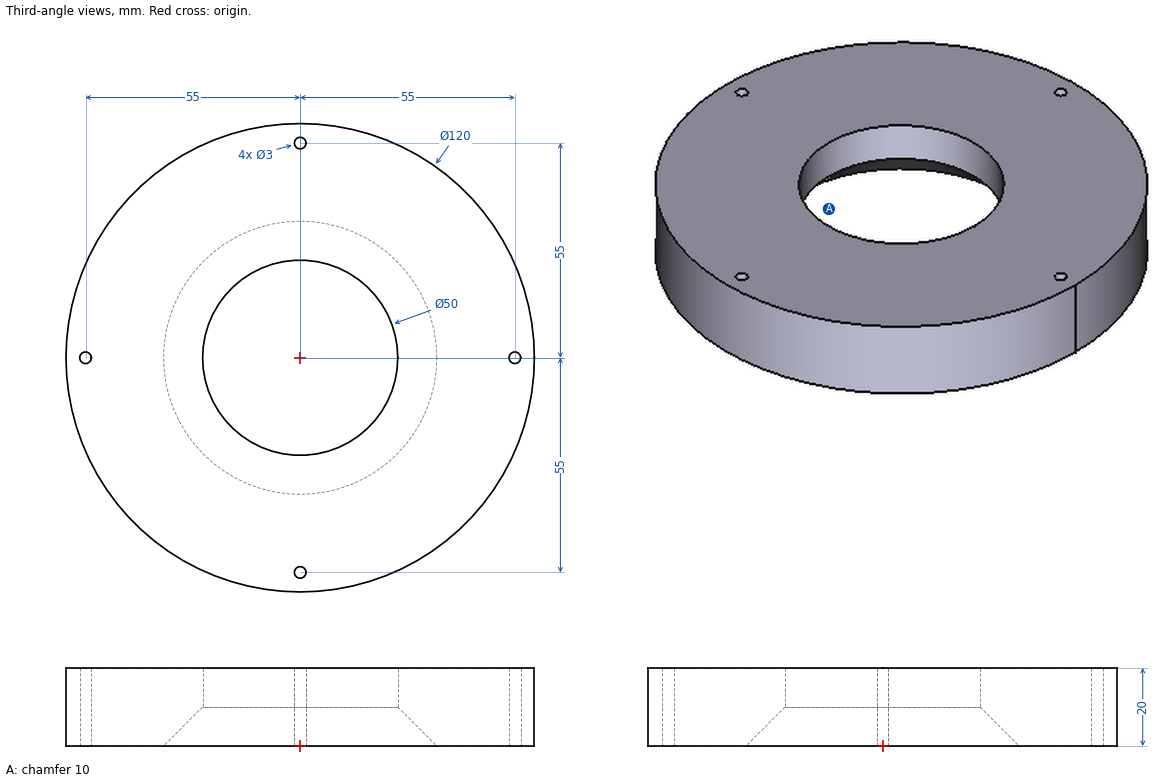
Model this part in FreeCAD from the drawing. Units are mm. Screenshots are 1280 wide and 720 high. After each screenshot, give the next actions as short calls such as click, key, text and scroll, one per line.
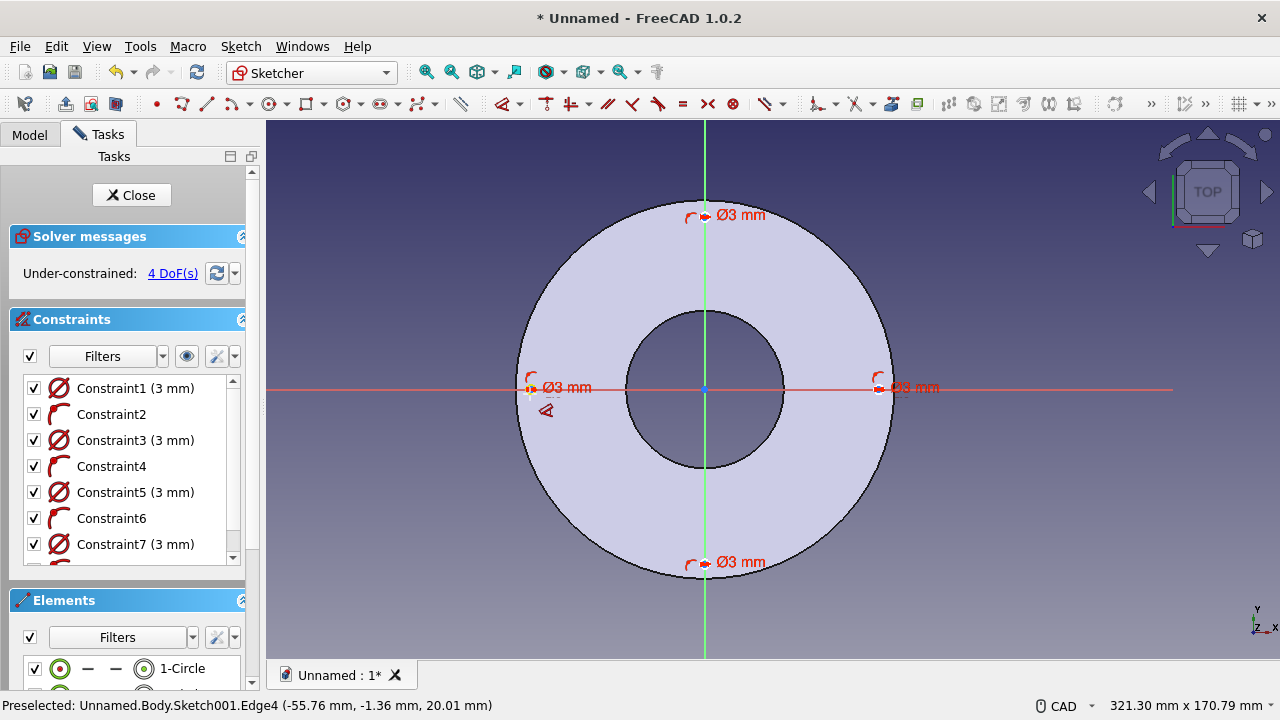
click(705, 217)
click(739, 303)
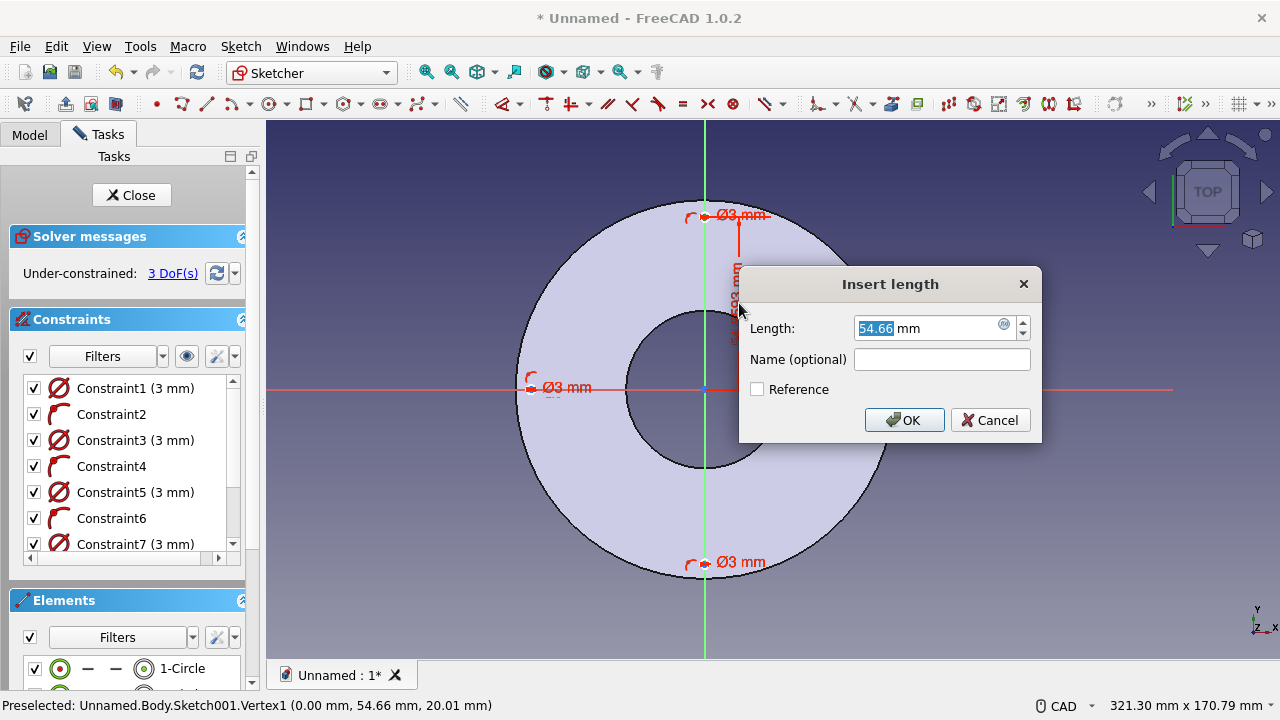
text(55)
key(Return)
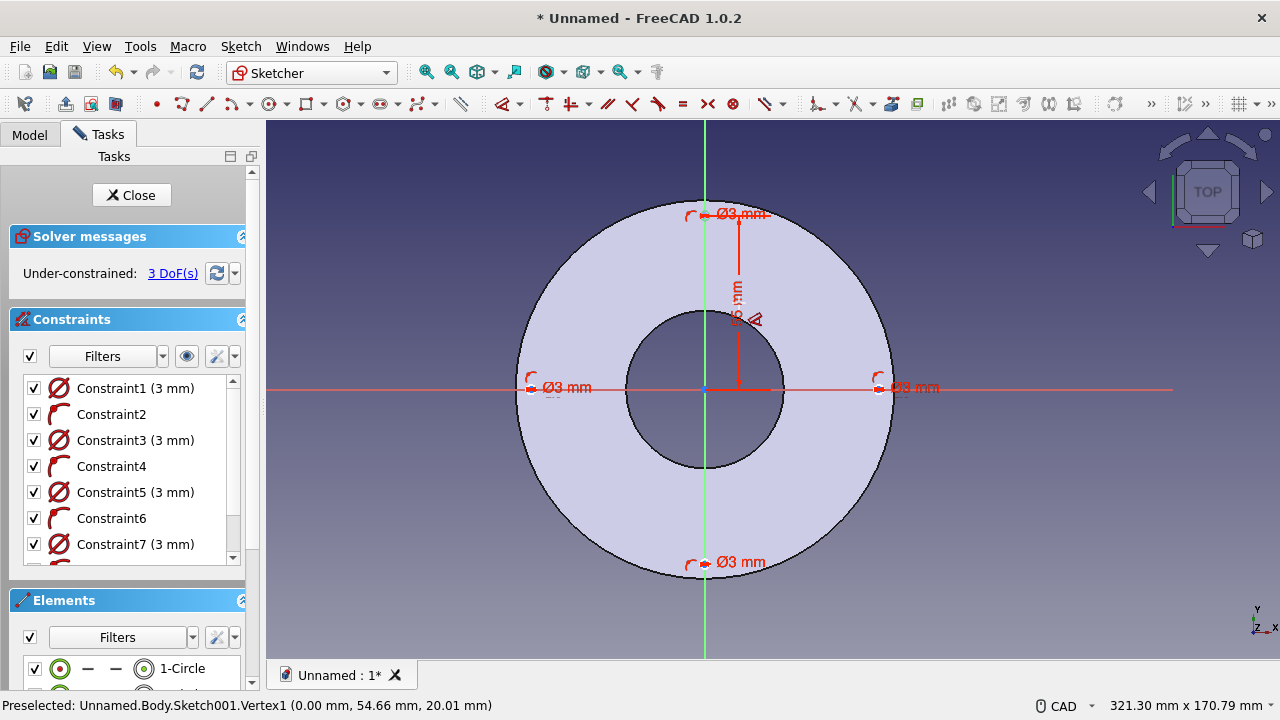
click(879, 390)
click(792, 424)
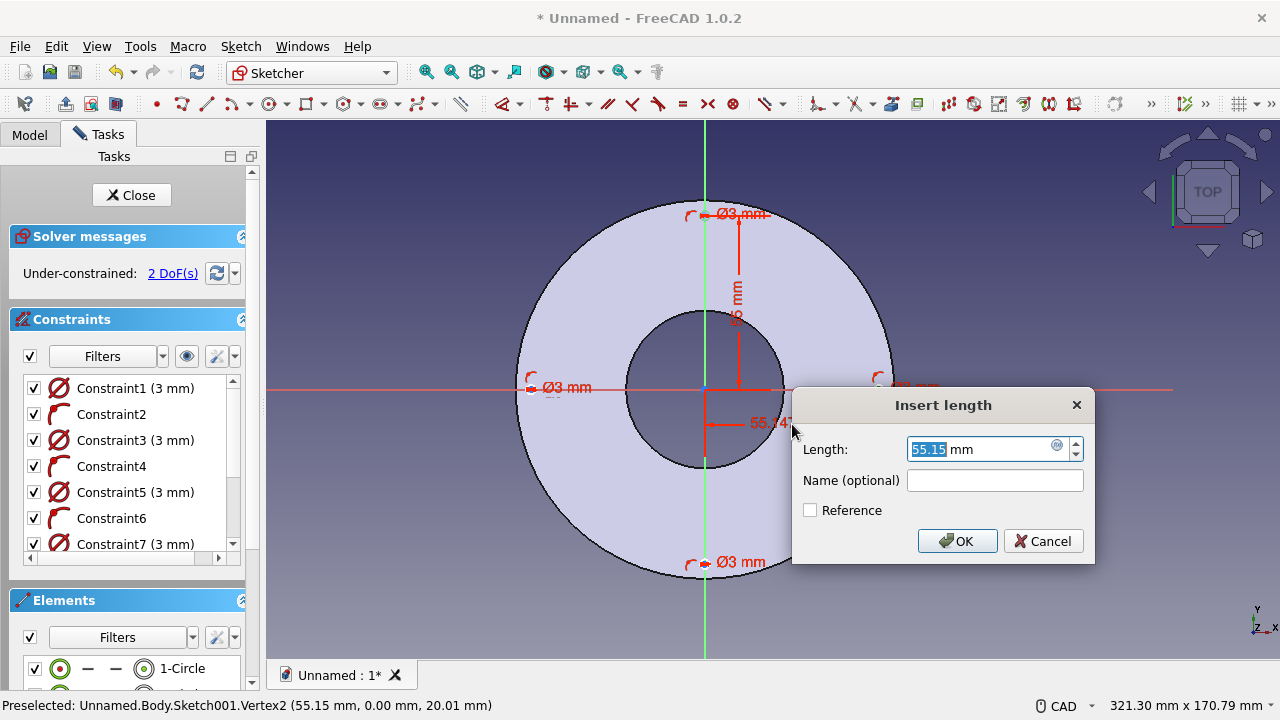
text(55)
key(Return)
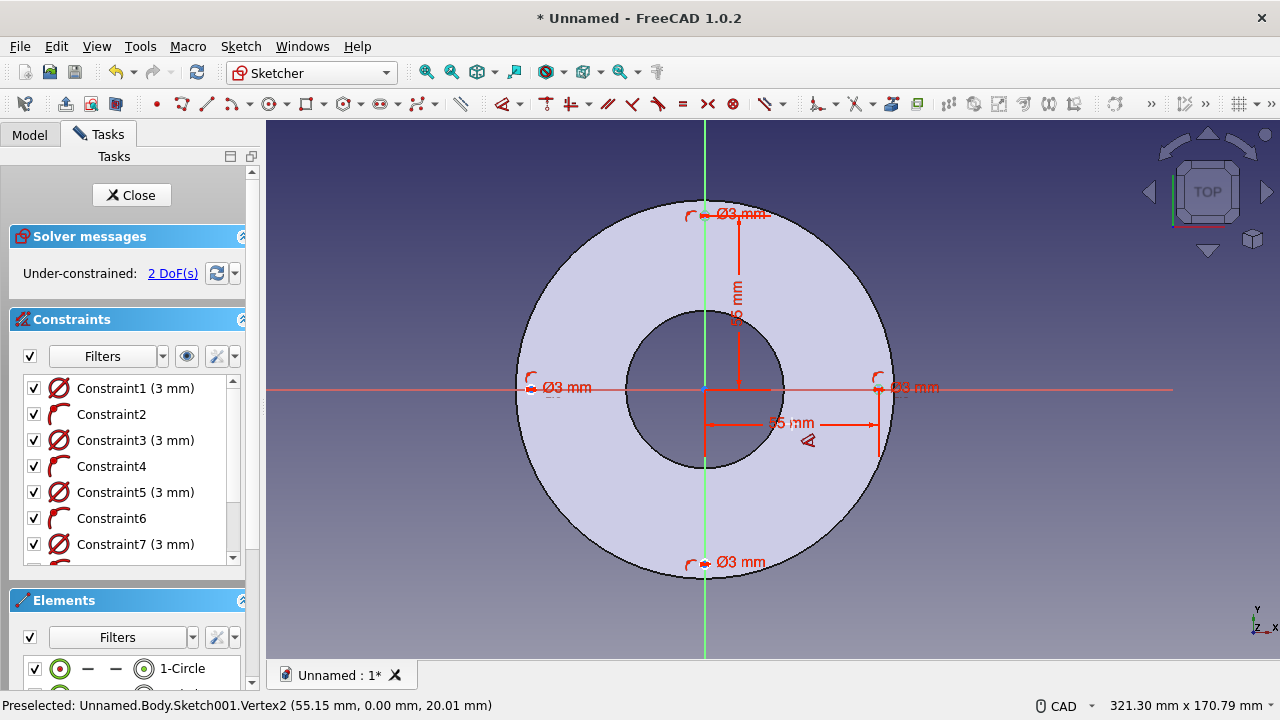
click(705, 564)
click(739, 477)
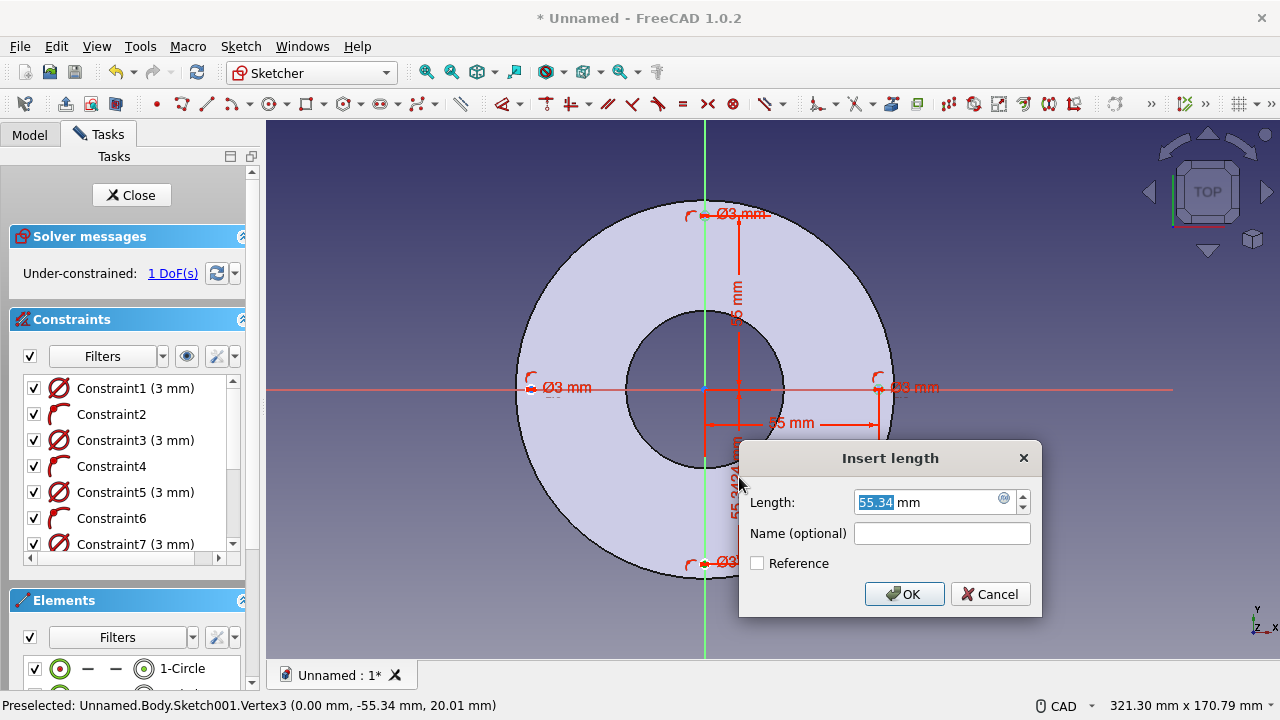
text(55)
key(Return)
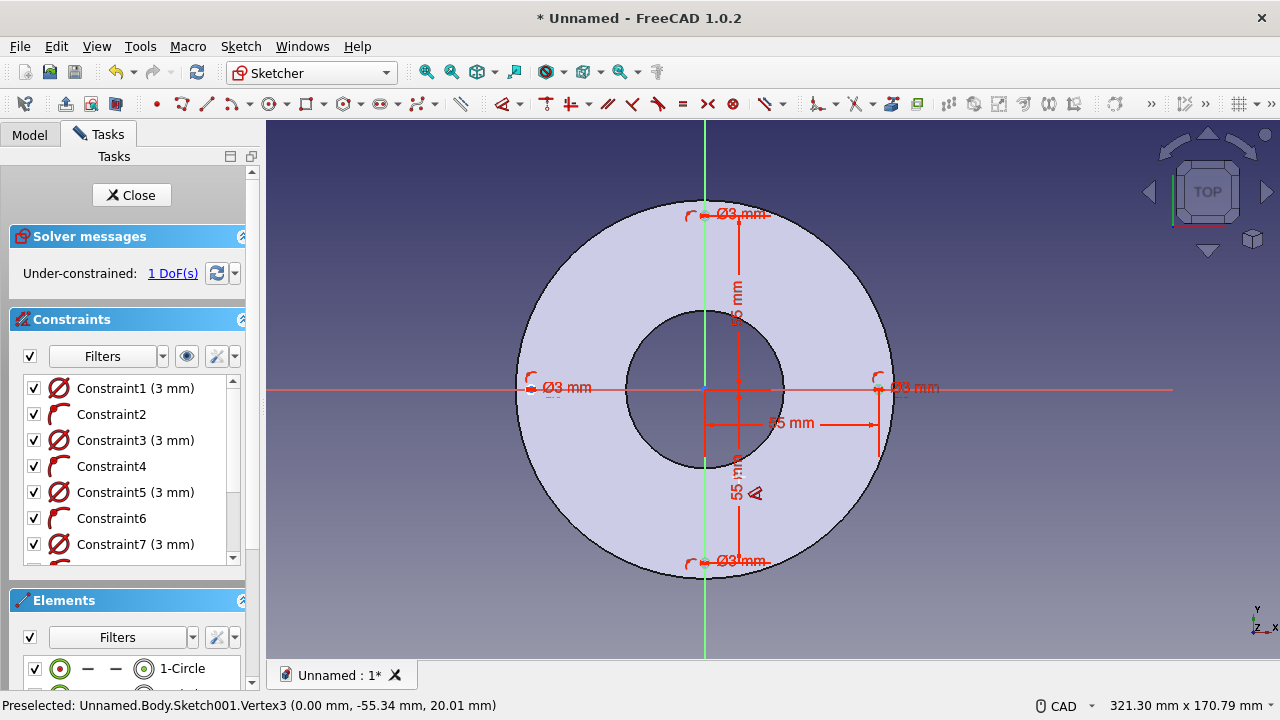
click(531, 390)
click(618, 424)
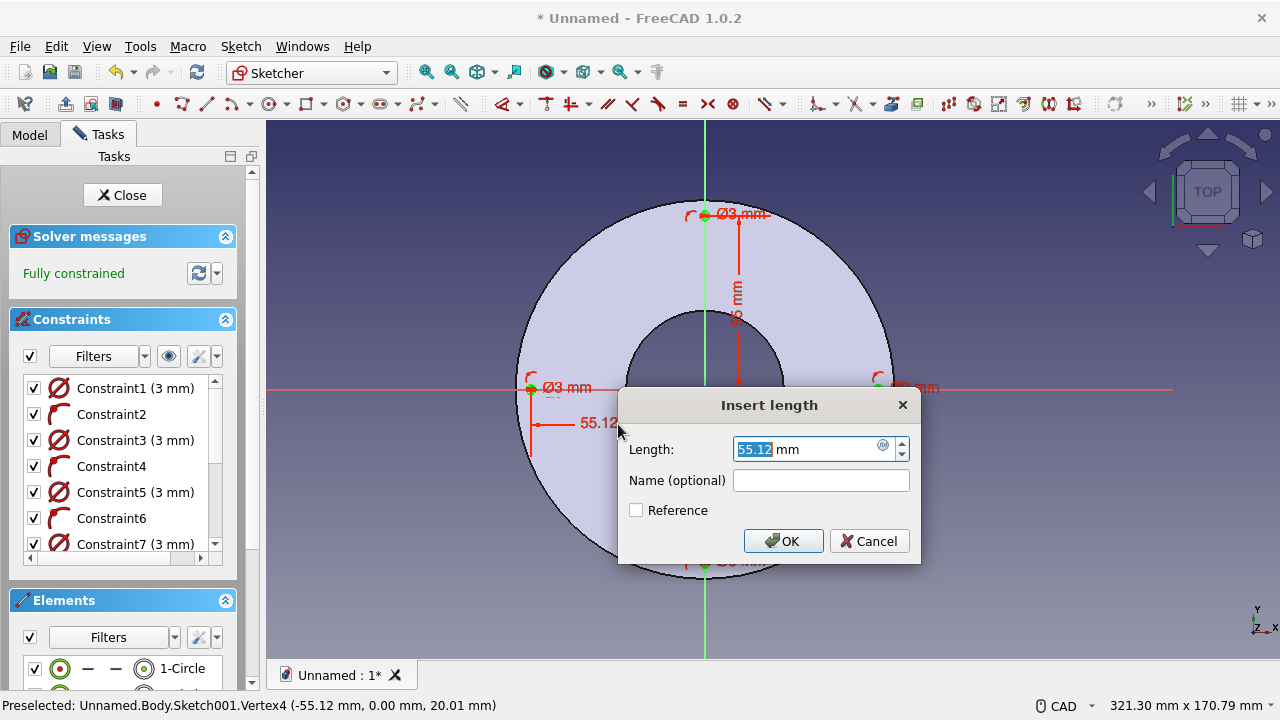
text(55)
key(Return)
key(Escape)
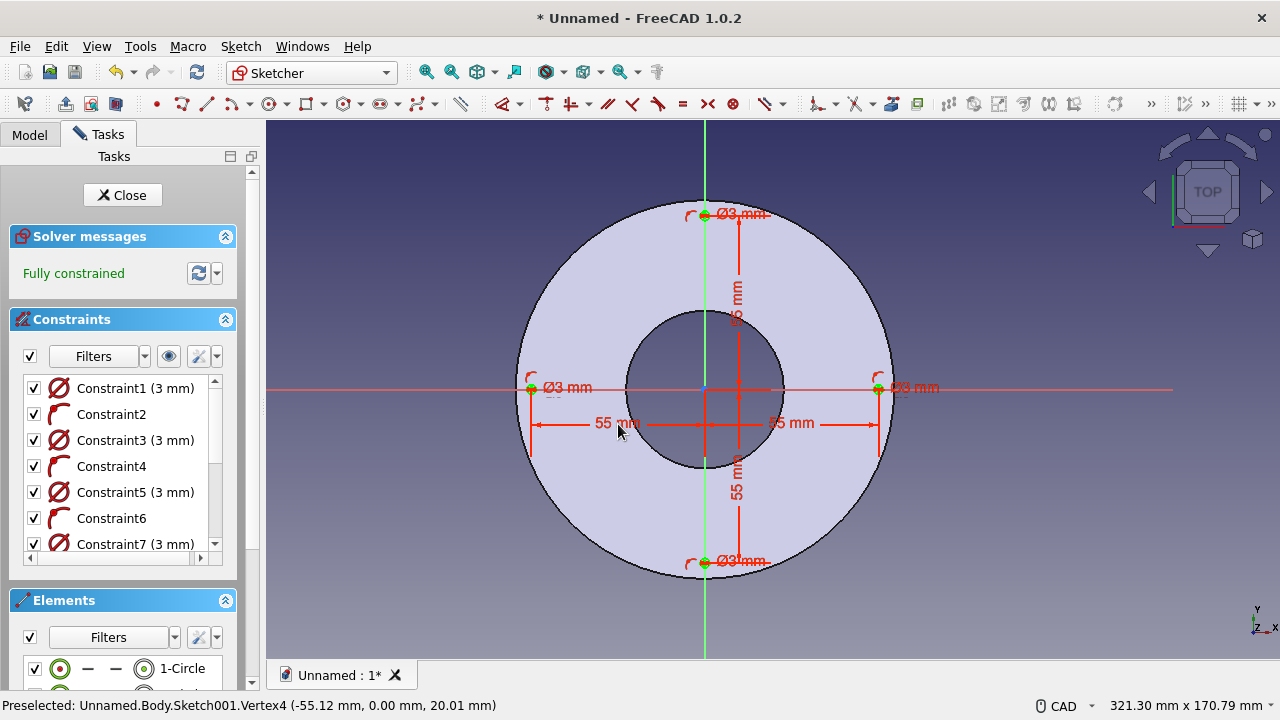
click(123, 195)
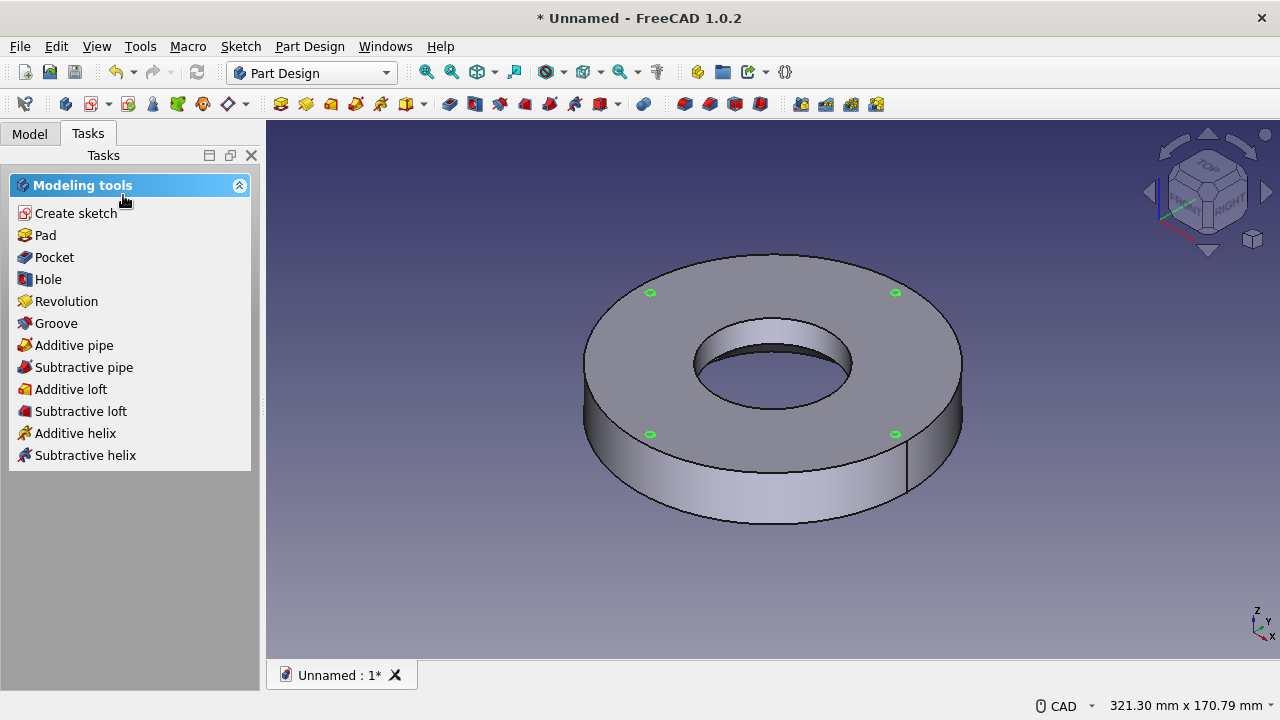
click(450, 104)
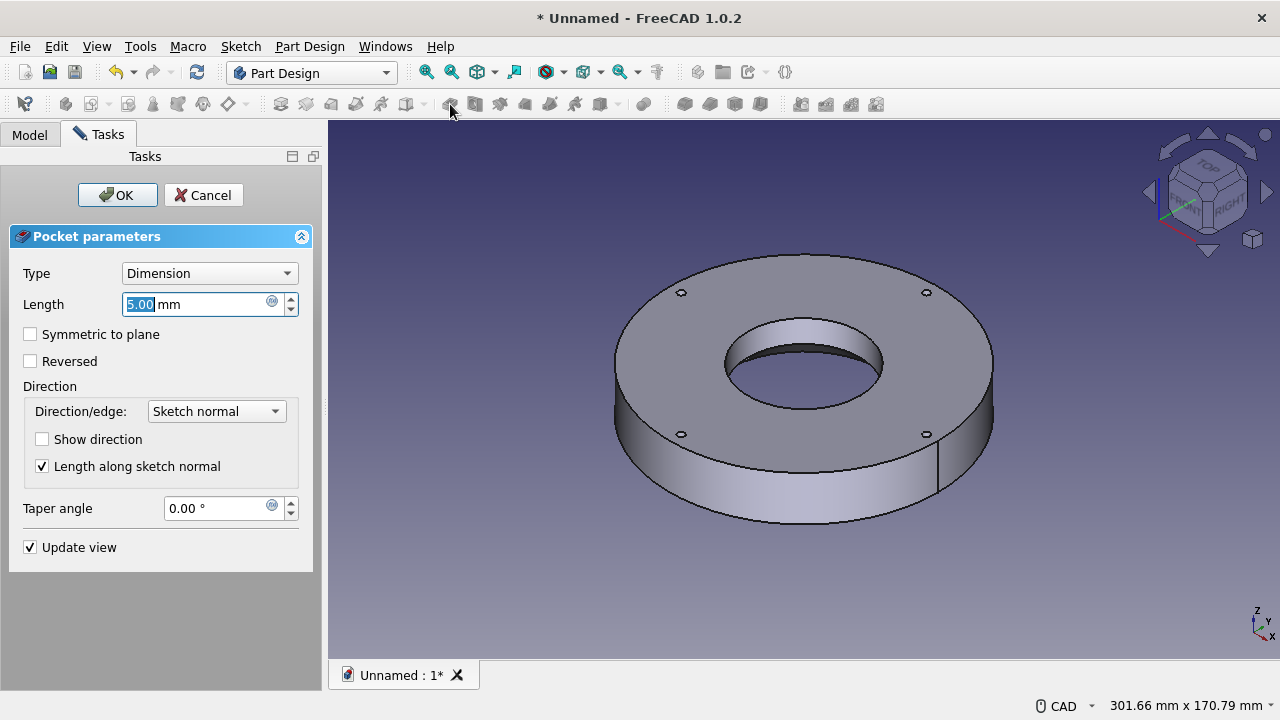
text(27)
key(Tab)